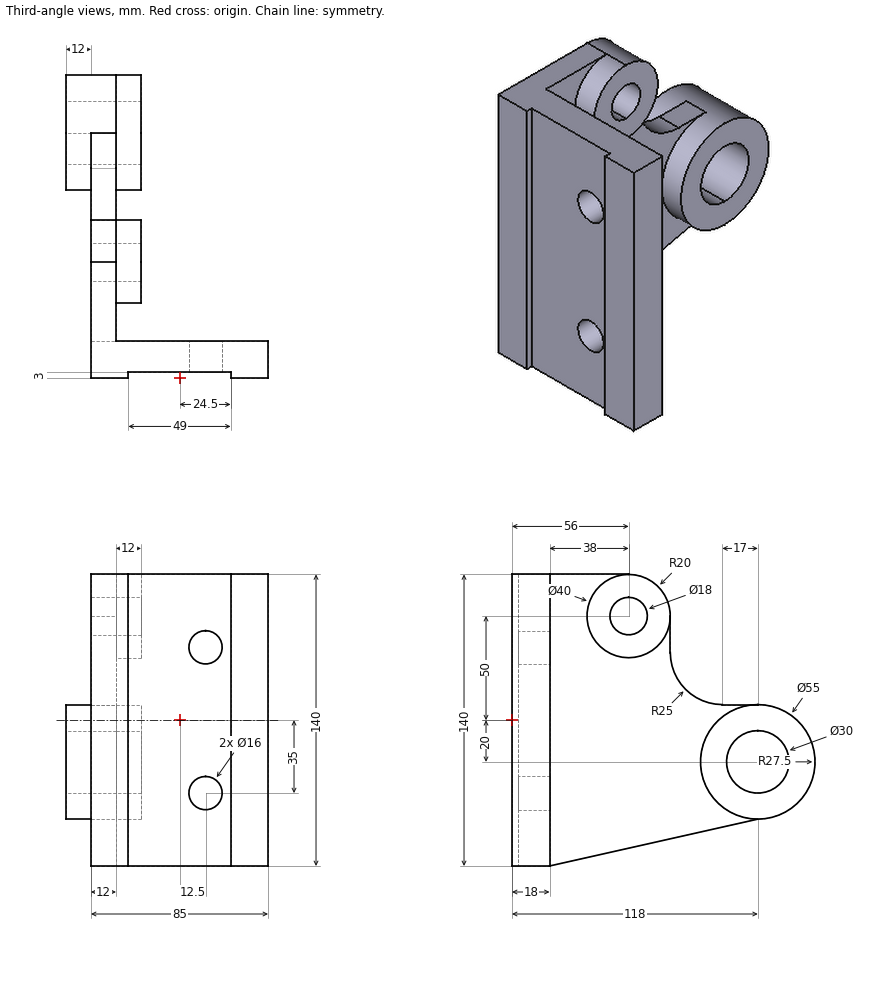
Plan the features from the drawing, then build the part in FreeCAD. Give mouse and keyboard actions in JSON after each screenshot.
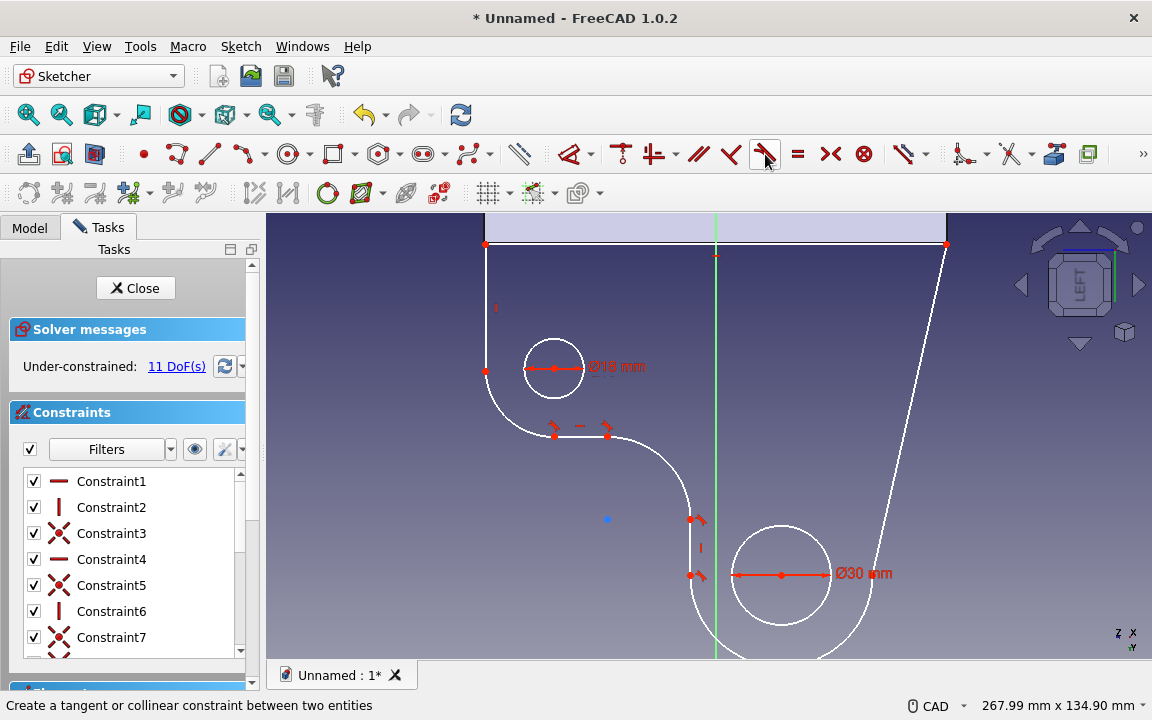
{"action": "left_click", "coordinate": [486, 282]}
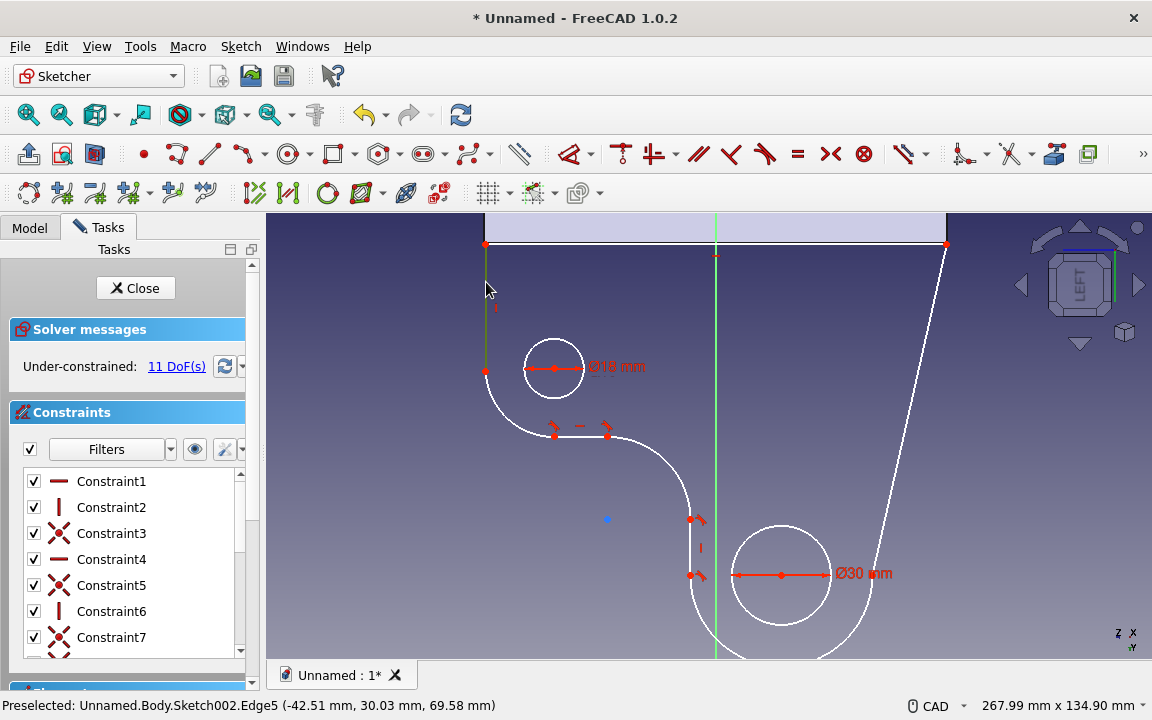
{"action": "left_click", "coordinate": [494, 401]}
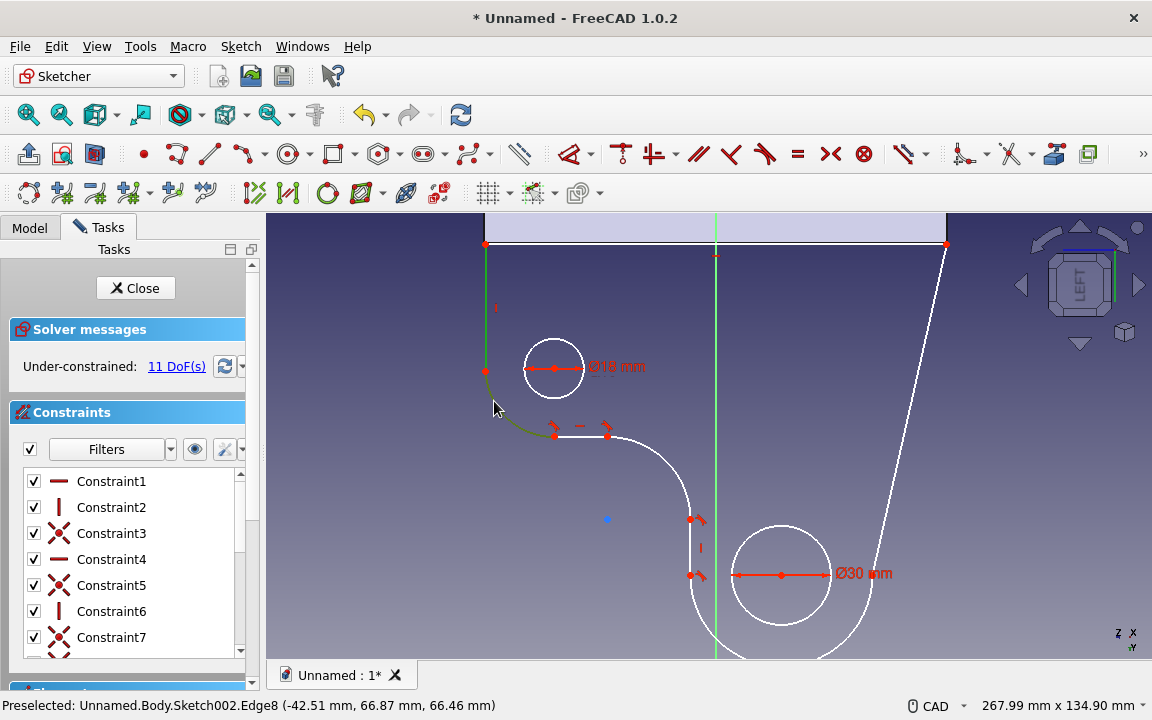
{"action": "left_click", "coordinate": [765, 154]}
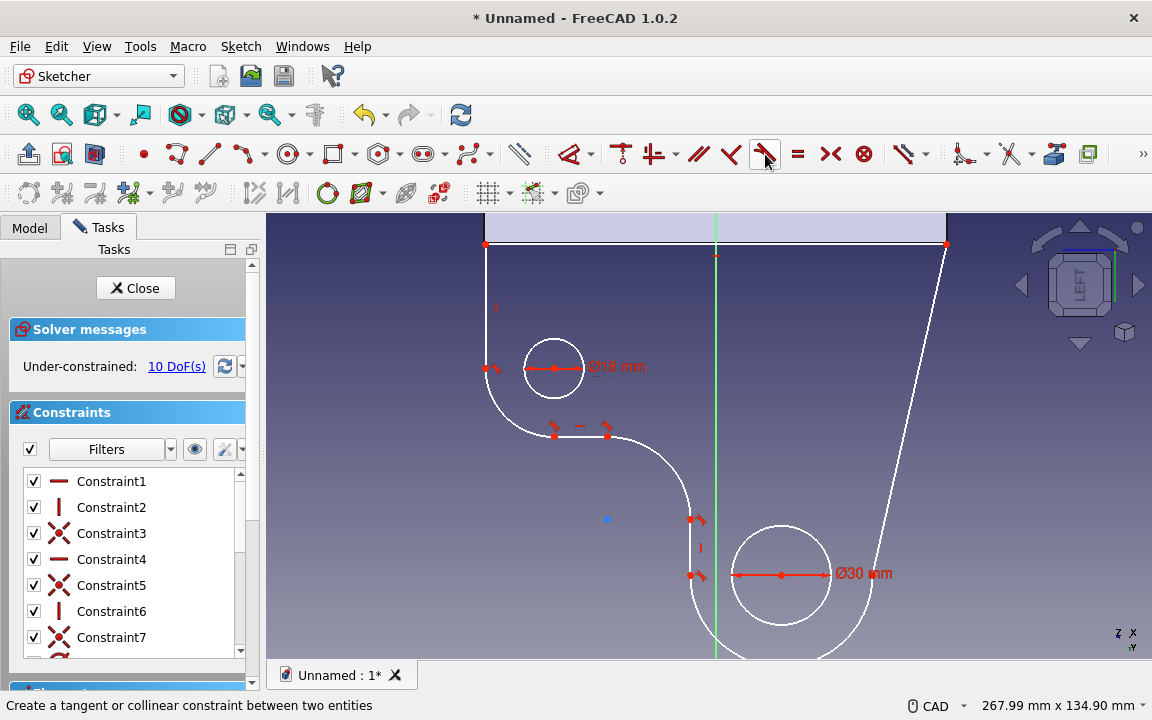
{"action": "key", "text": "d"}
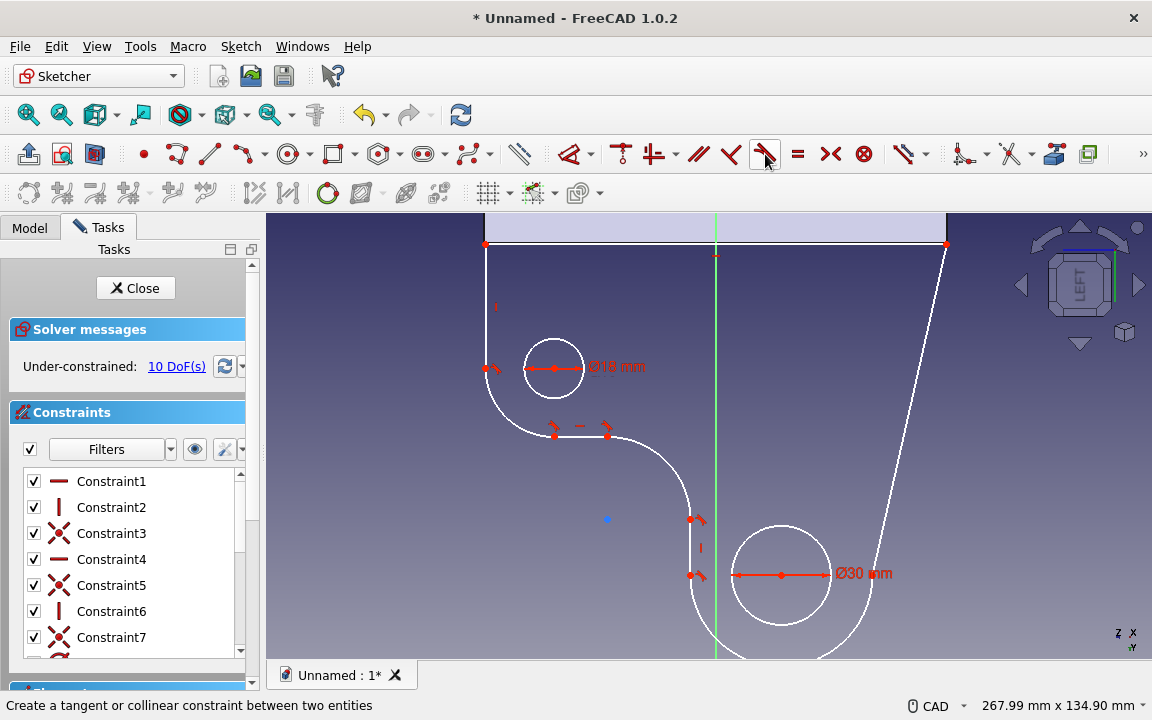
{"action": "left_click", "coordinate": [681, 482]}
{"action": "left_click", "coordinate": [672, 425]}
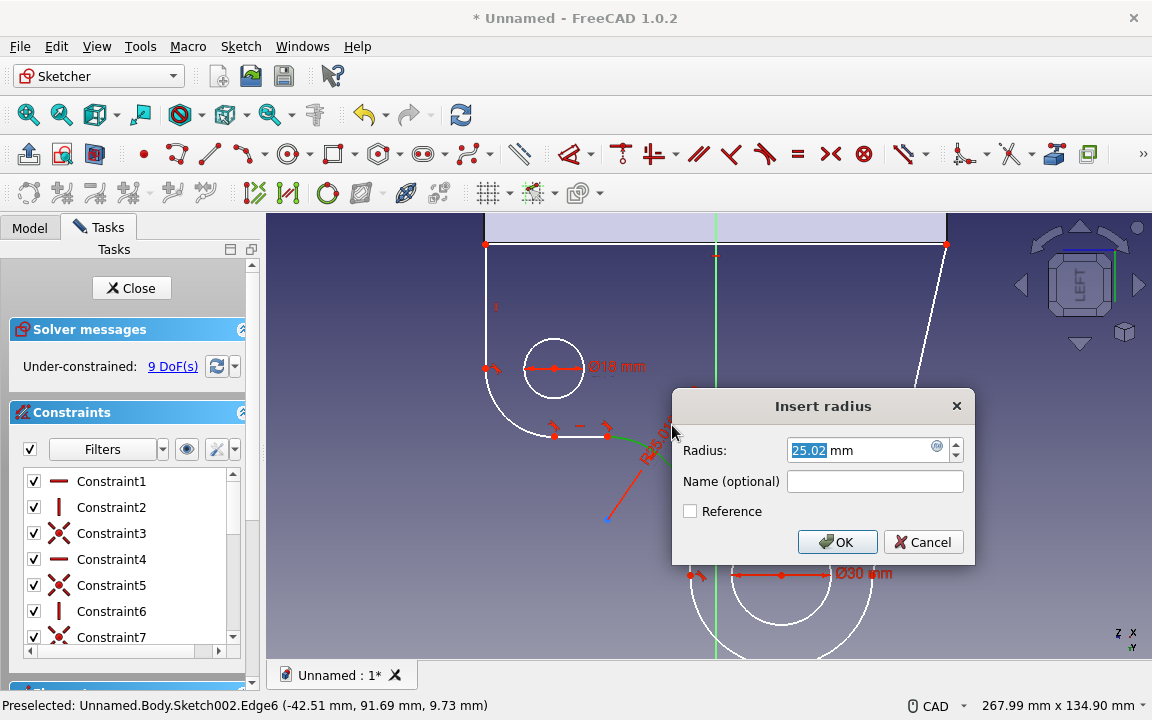
{"action": "type", "text": "25"}
{"action": "key", "text": "Return"}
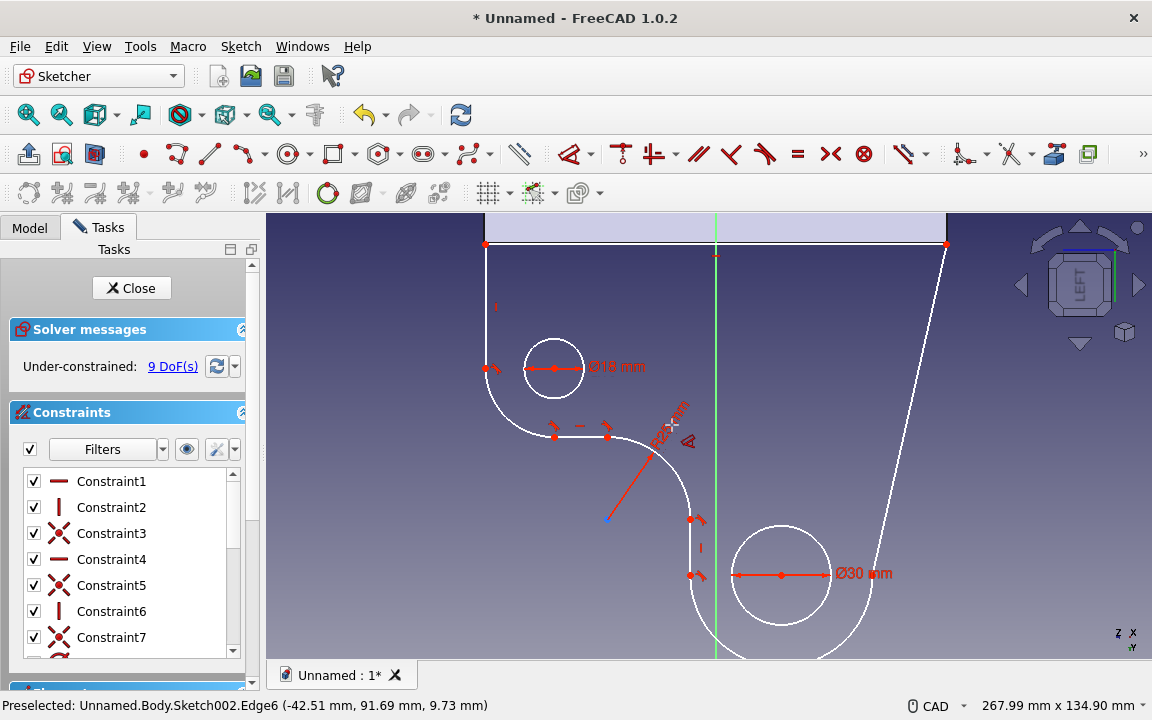
{"action": "left_click", "coordinate": [855, 629]}
{"action": "left_click", "coordinate": [903, 591]}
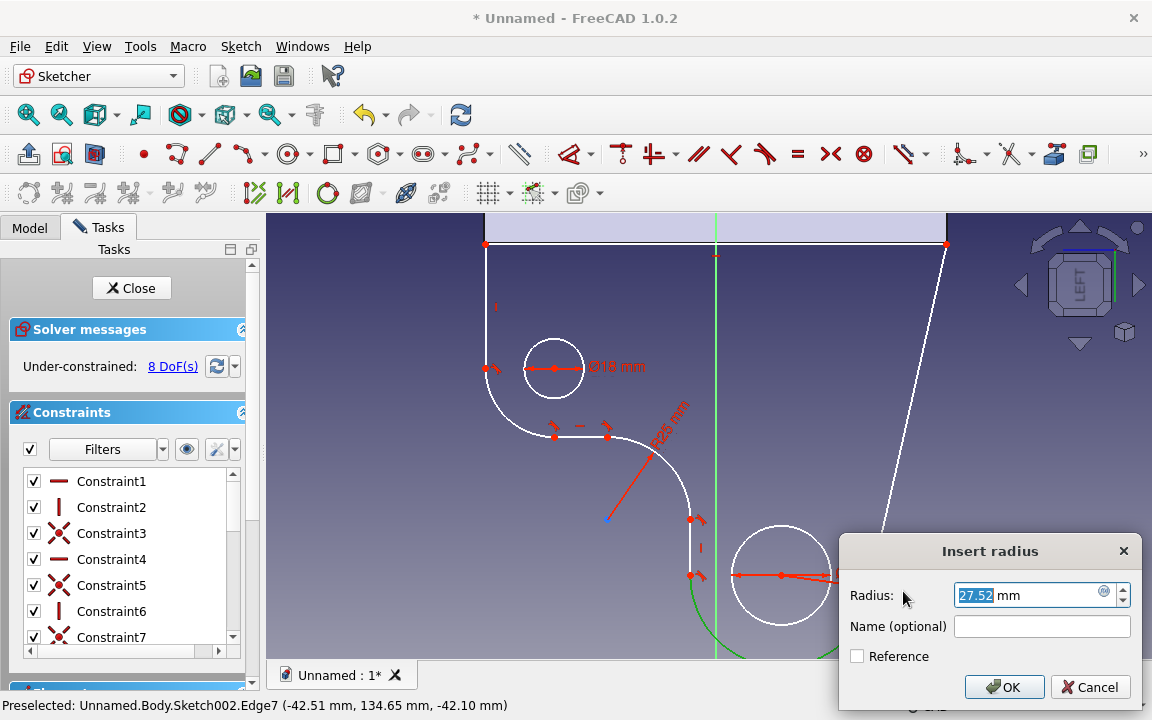
{"action": "type", "text": "27.5"}
{"action": "key", "text": "Return"}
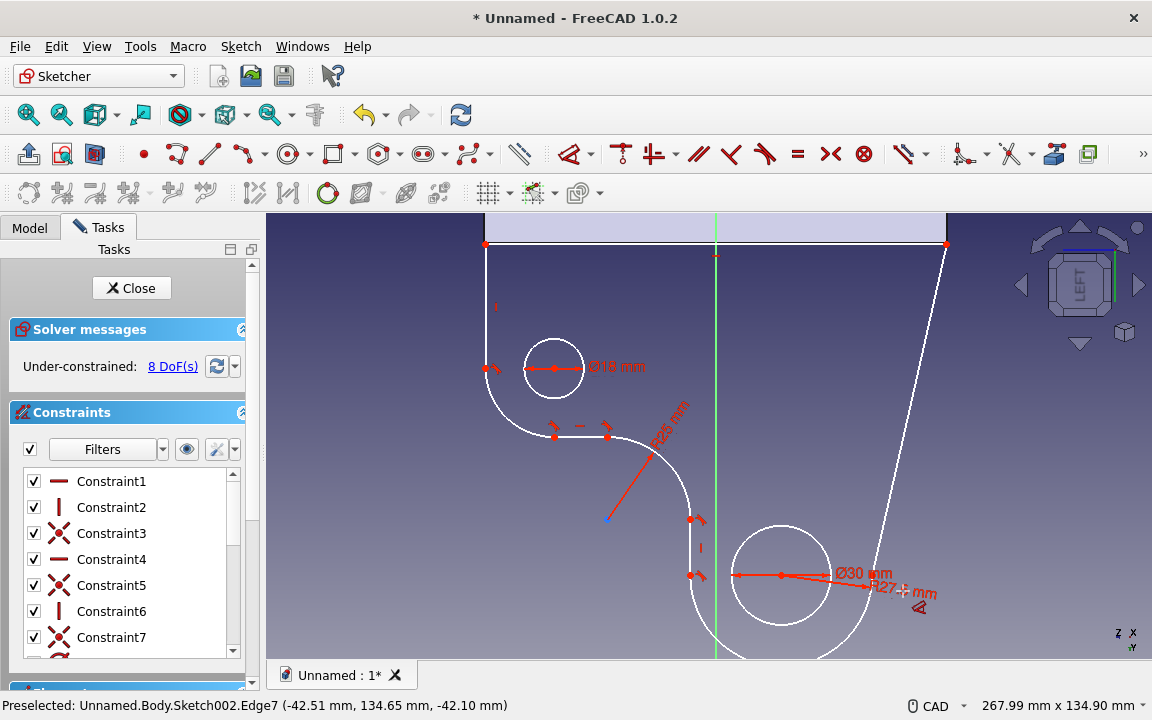
{"action": "left_click", "coordinate": [493, 400]}
{"action": "left_click", "coordinate": [465, 415]}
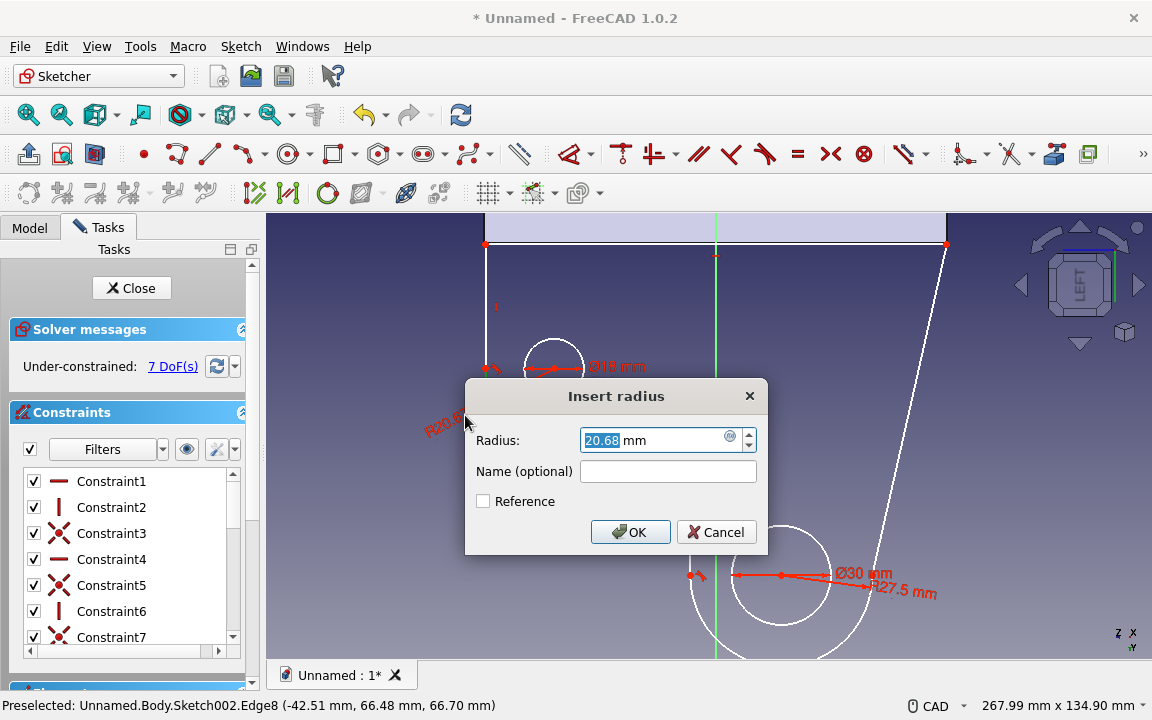
{"action": "type", "text": "20"}
{"action": "key", "text": "Return"}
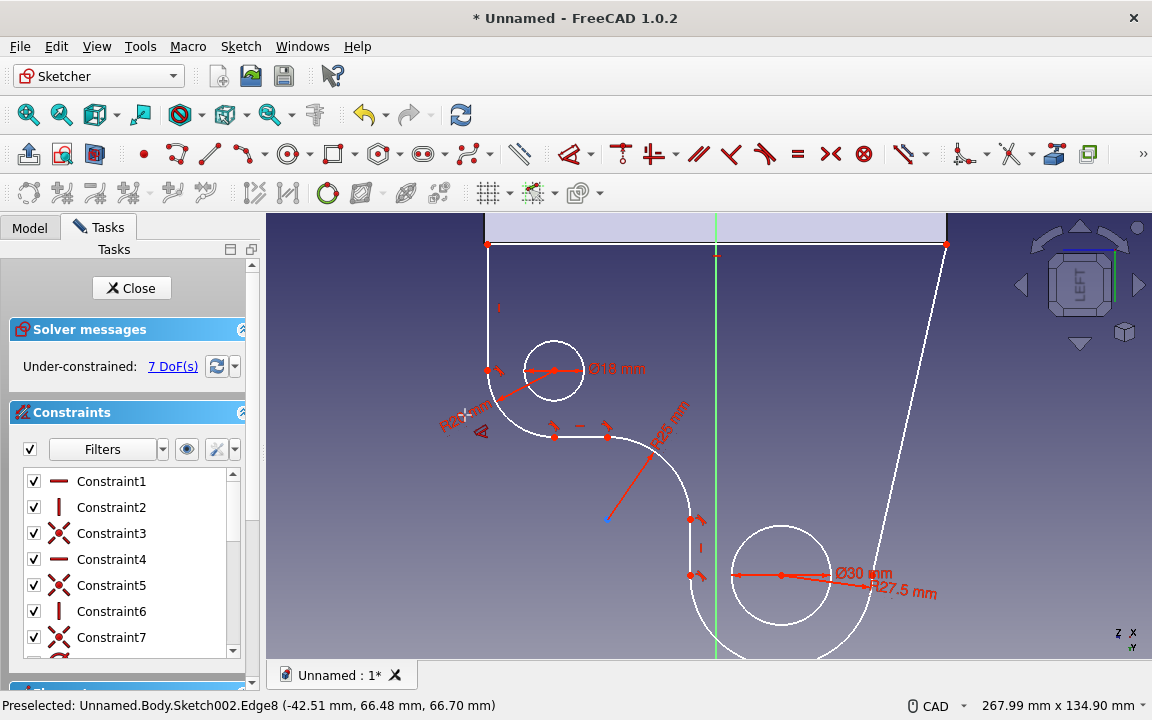
{"action": "left_click", "coordinate": [690, 536]}
{"action": "left_click", "coordinate": [656, 548]}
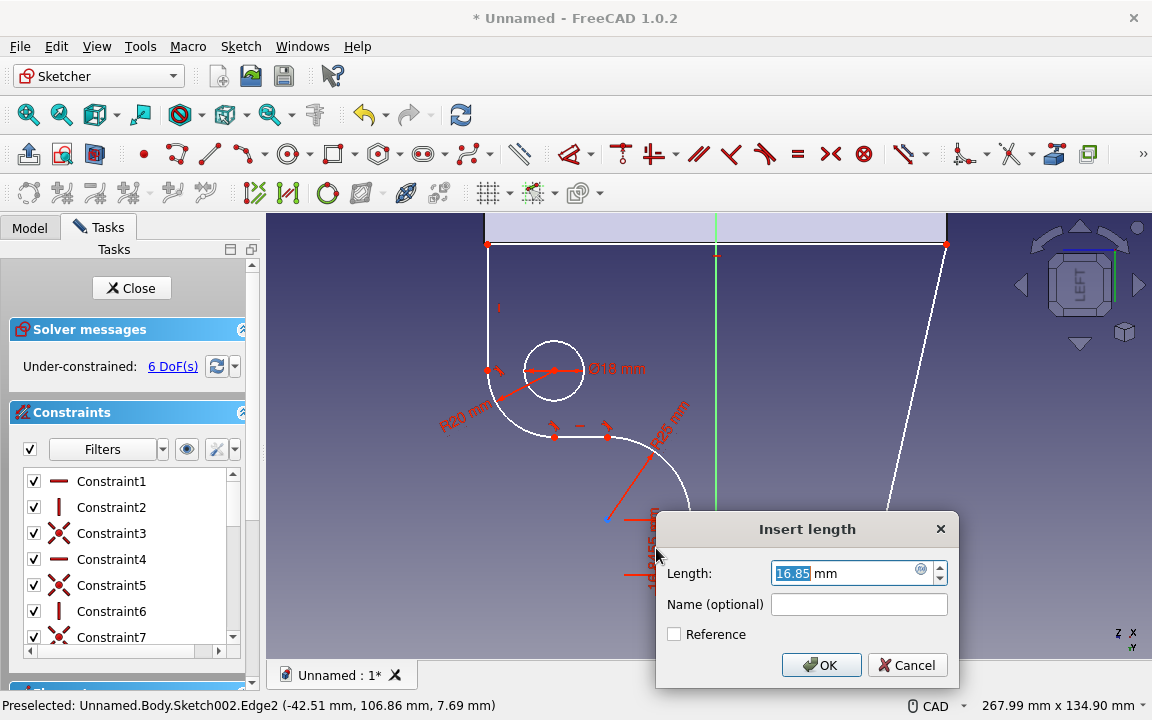
{"action": "type", "text": "17"}
{"action": "key", "text": "Return"}